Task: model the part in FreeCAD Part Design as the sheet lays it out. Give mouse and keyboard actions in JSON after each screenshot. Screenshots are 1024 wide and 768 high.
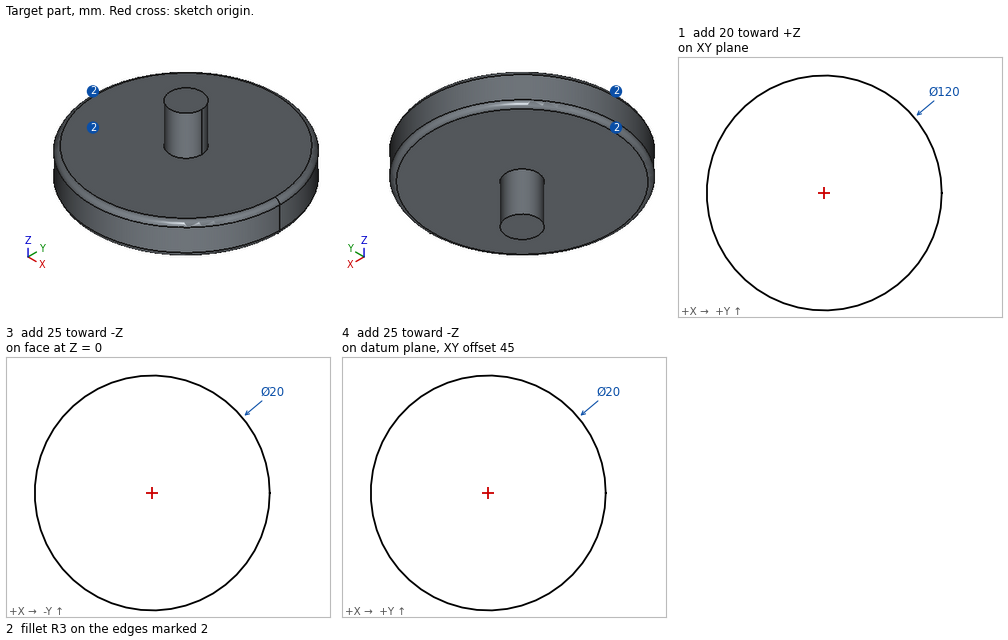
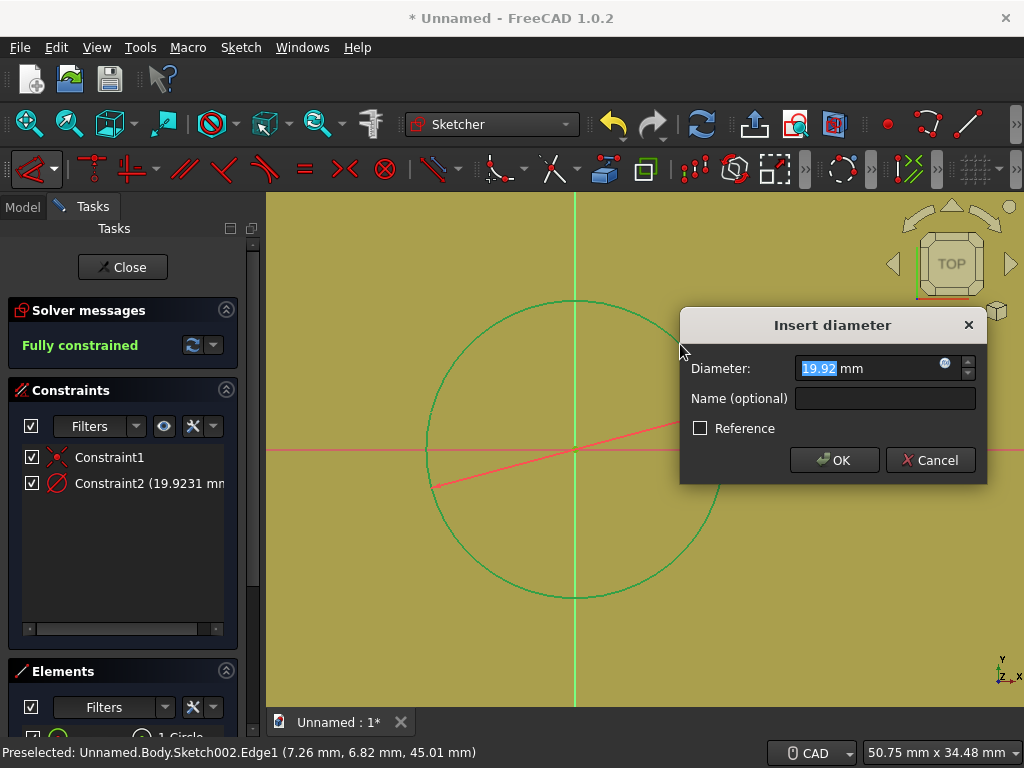
{"action": "type", "text": "20"}
{"action": "key", "text": "Return"}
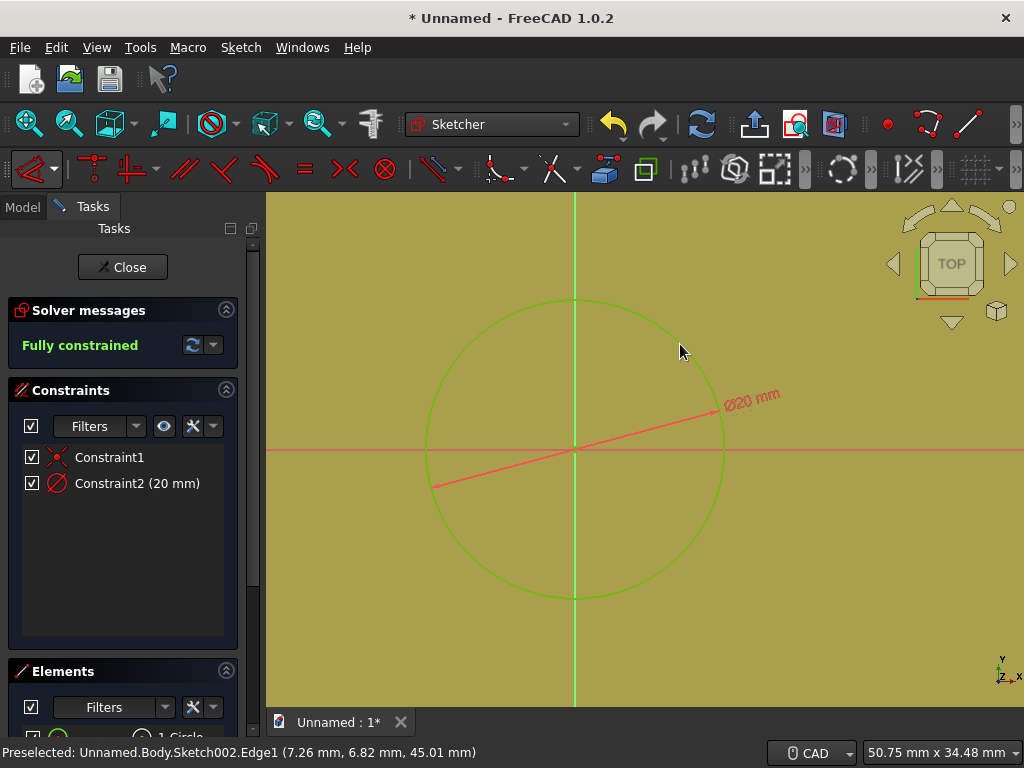
{"action": "left_click", "coordinate": [123, 267]}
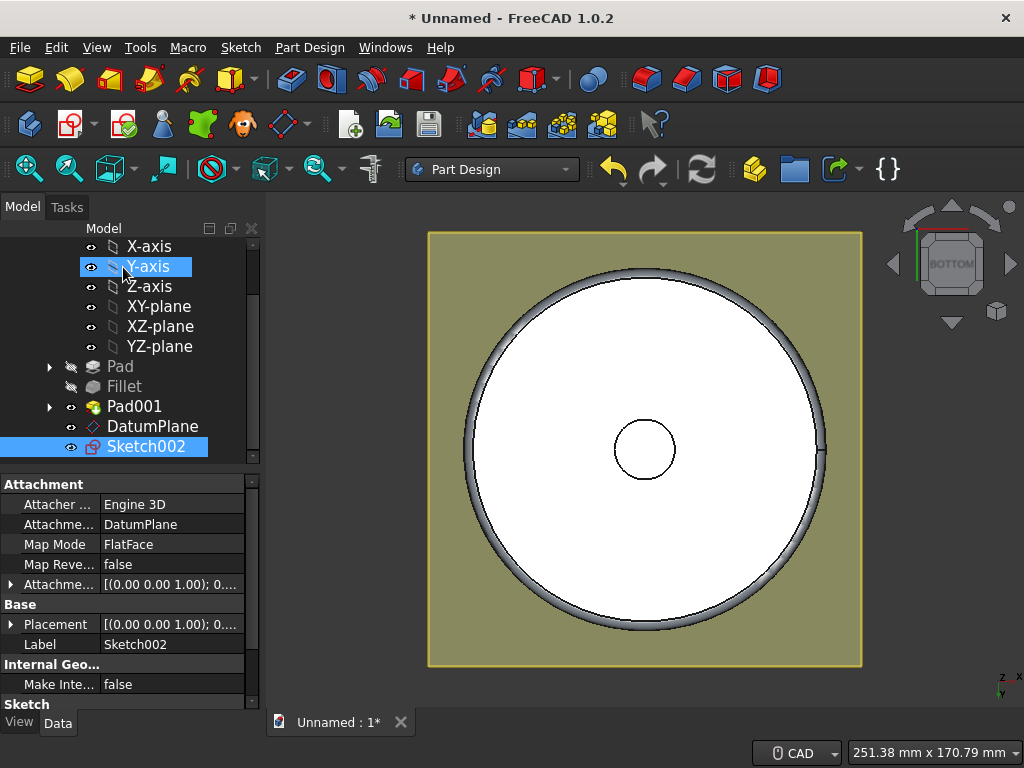
{"action": "left_click", "coordinate": [30, 80]}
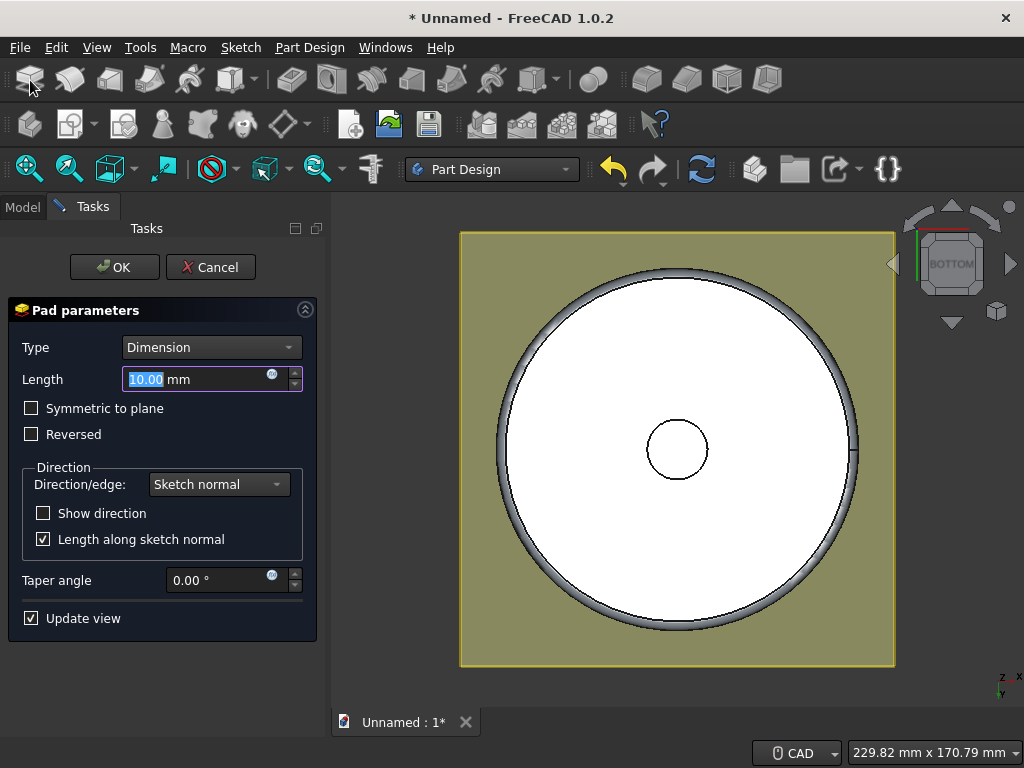
{"action": "type", "text": "25"}
{"action": "key", "text": "Tab"}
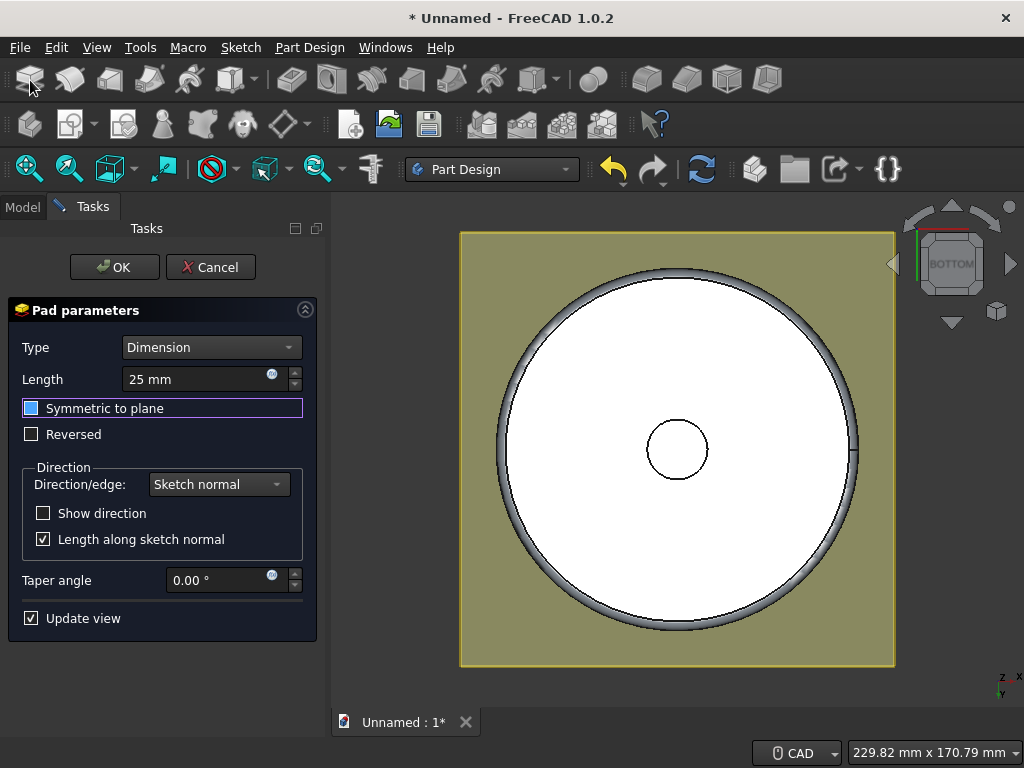
{"action": "left_click", "coordinate": [30, 434]}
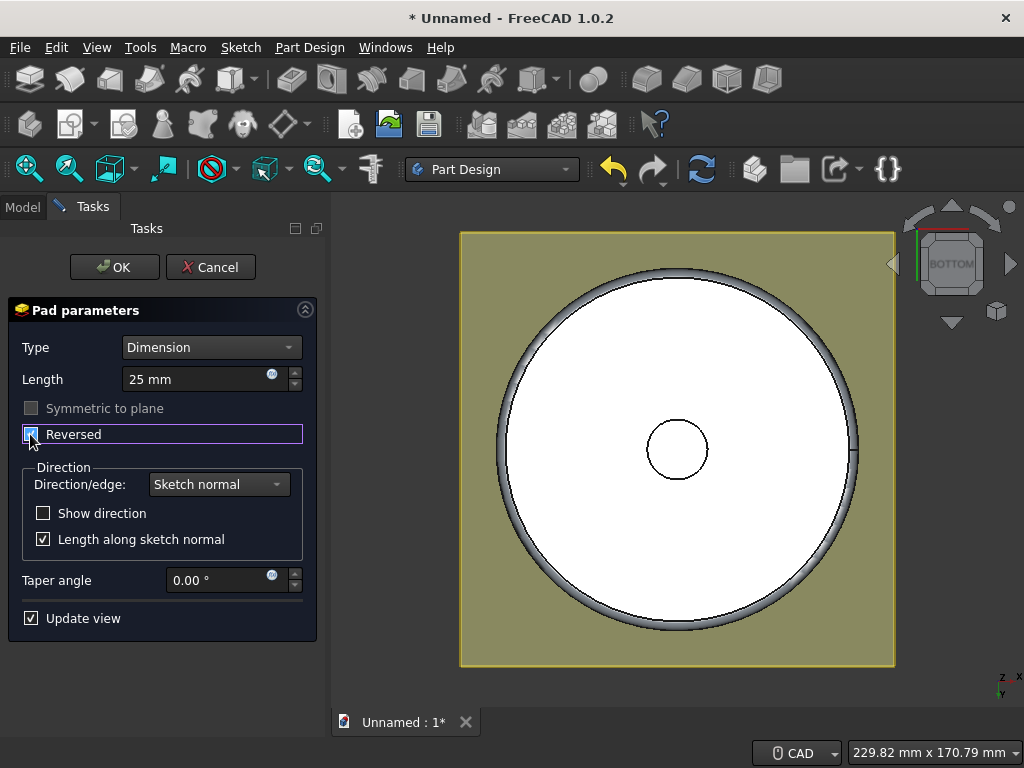
{"action": "left_click", "coordinate": [115, 267]}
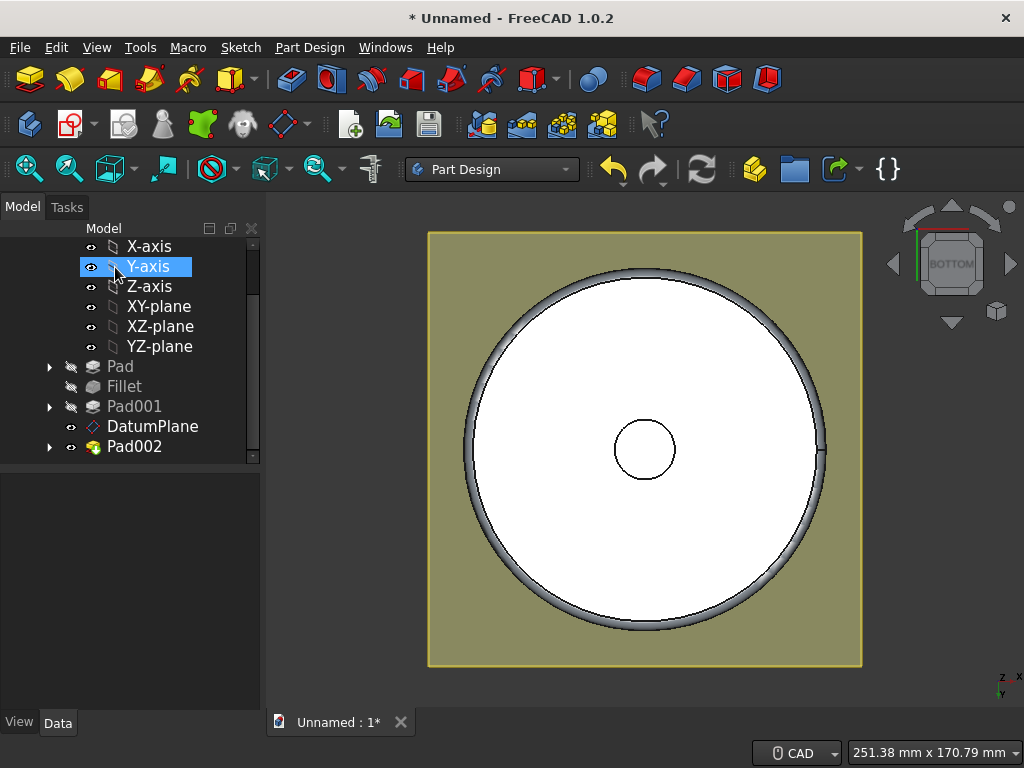
{"action": "left_click", "coordinate": [116, 427]}
{"action": "key", "text": "space"}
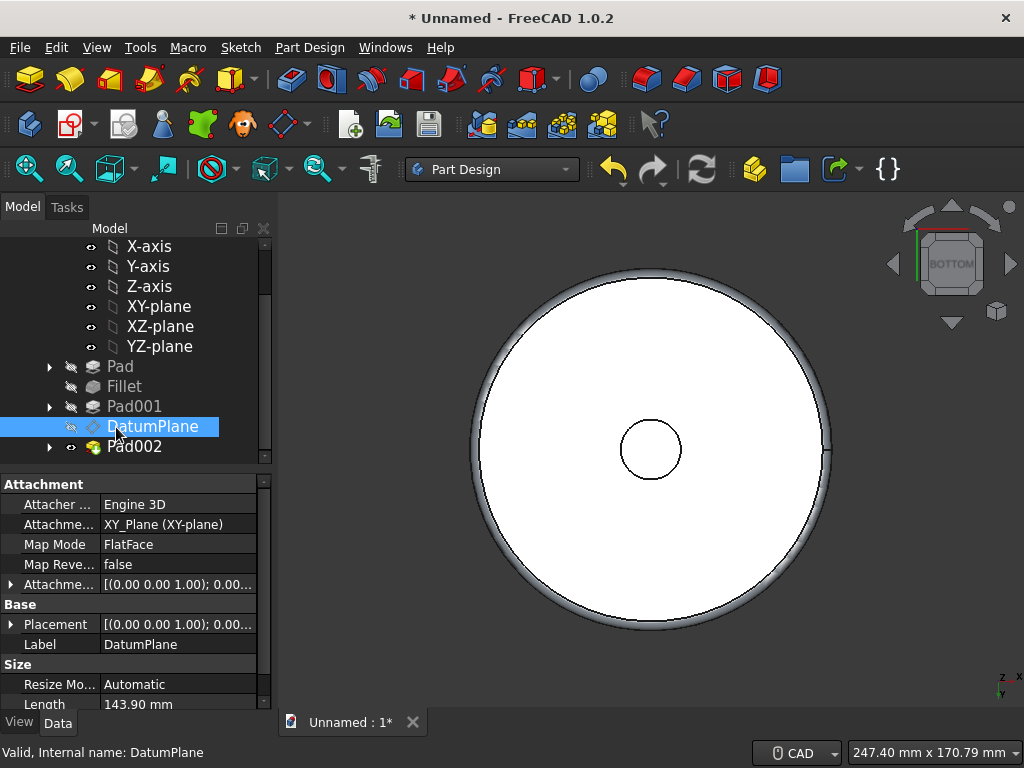
{"action": "key", "text": "0"}